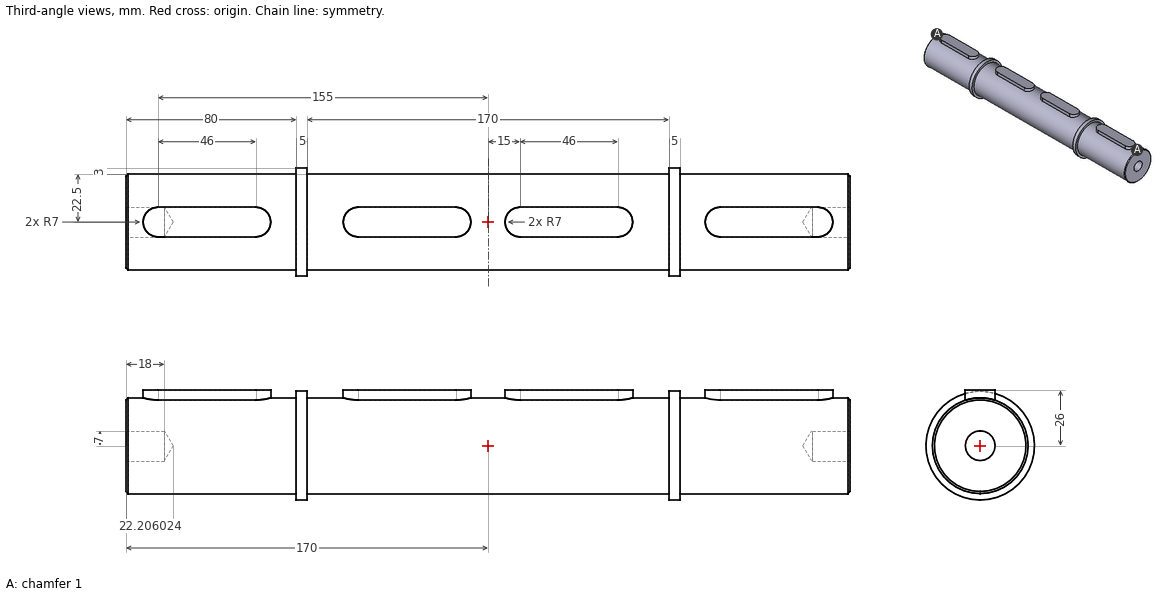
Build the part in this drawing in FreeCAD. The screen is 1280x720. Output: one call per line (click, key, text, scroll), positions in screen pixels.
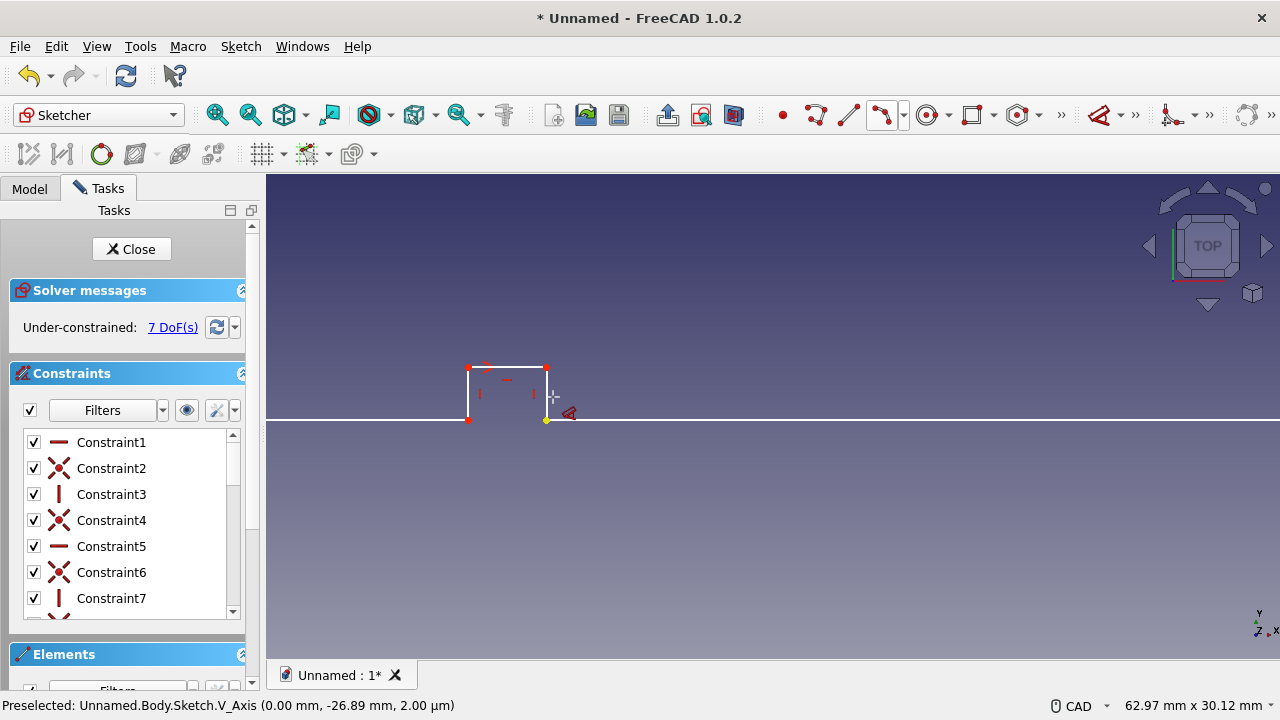
click(547, 394)
click(513, 394)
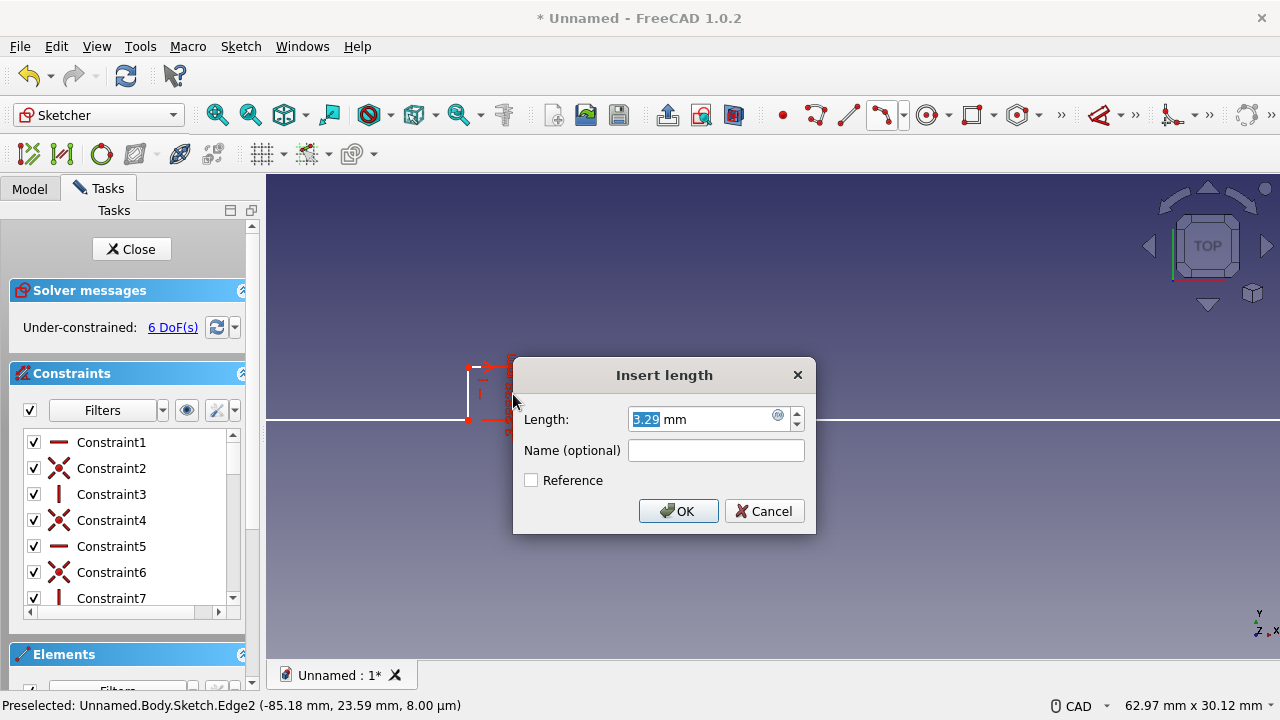
text(3)
key(Return)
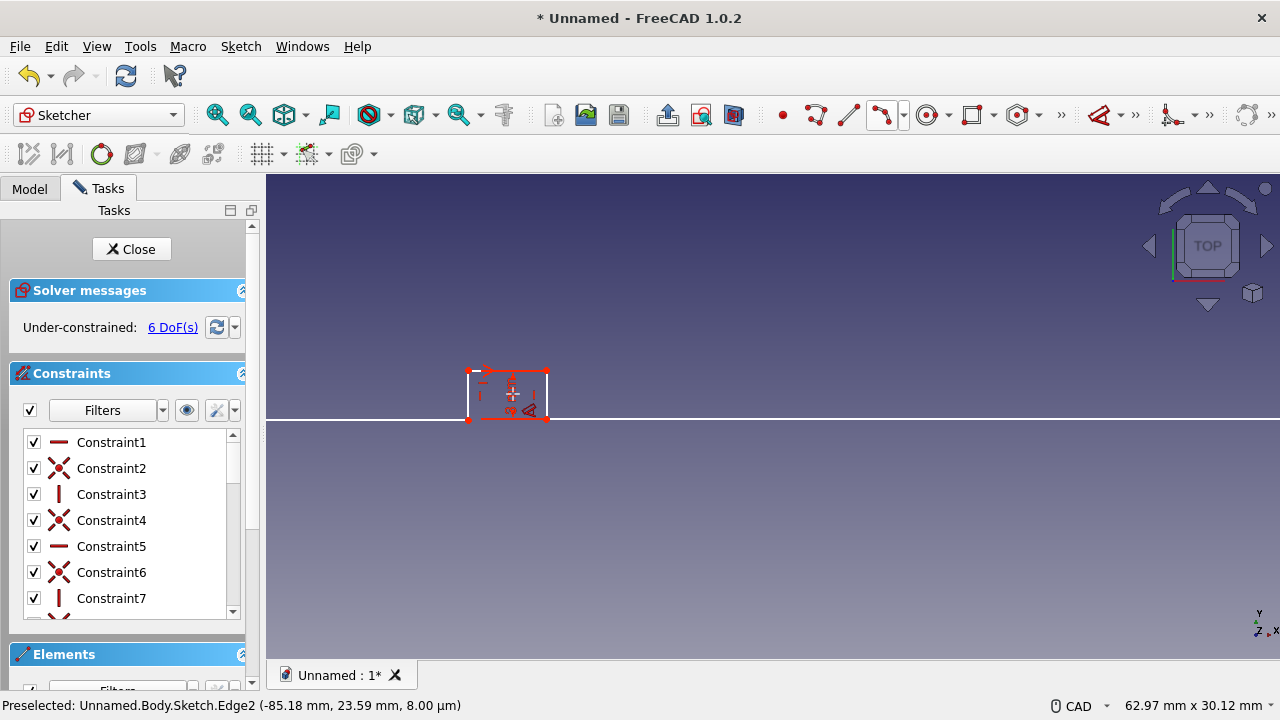
click(523, 371)
click(508, 337)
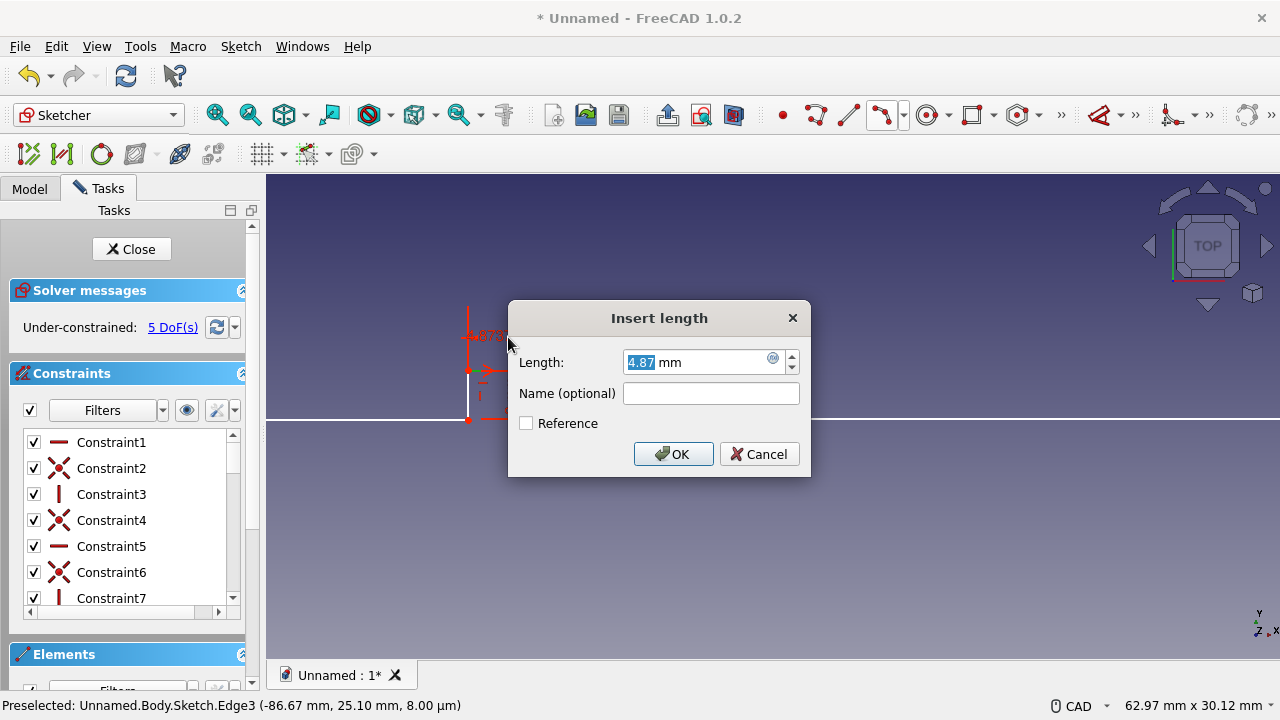
text(5)
key(Return)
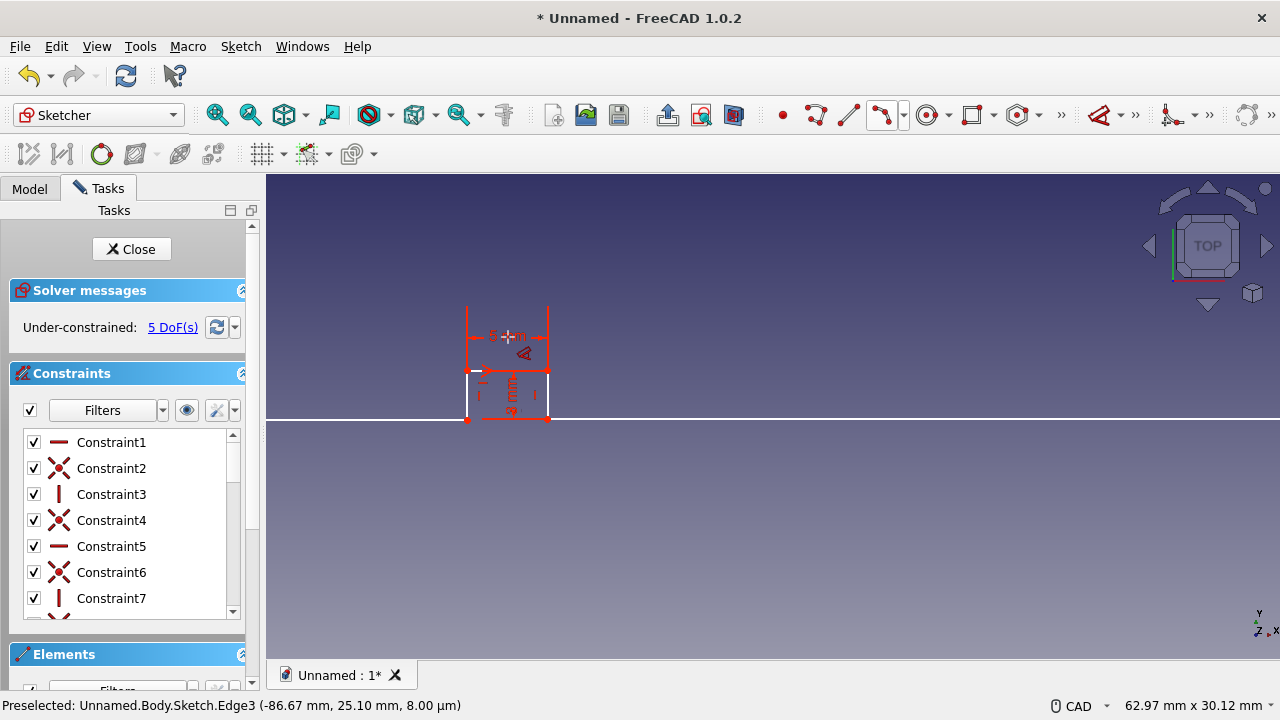
click(467, 386)
click(433, 395)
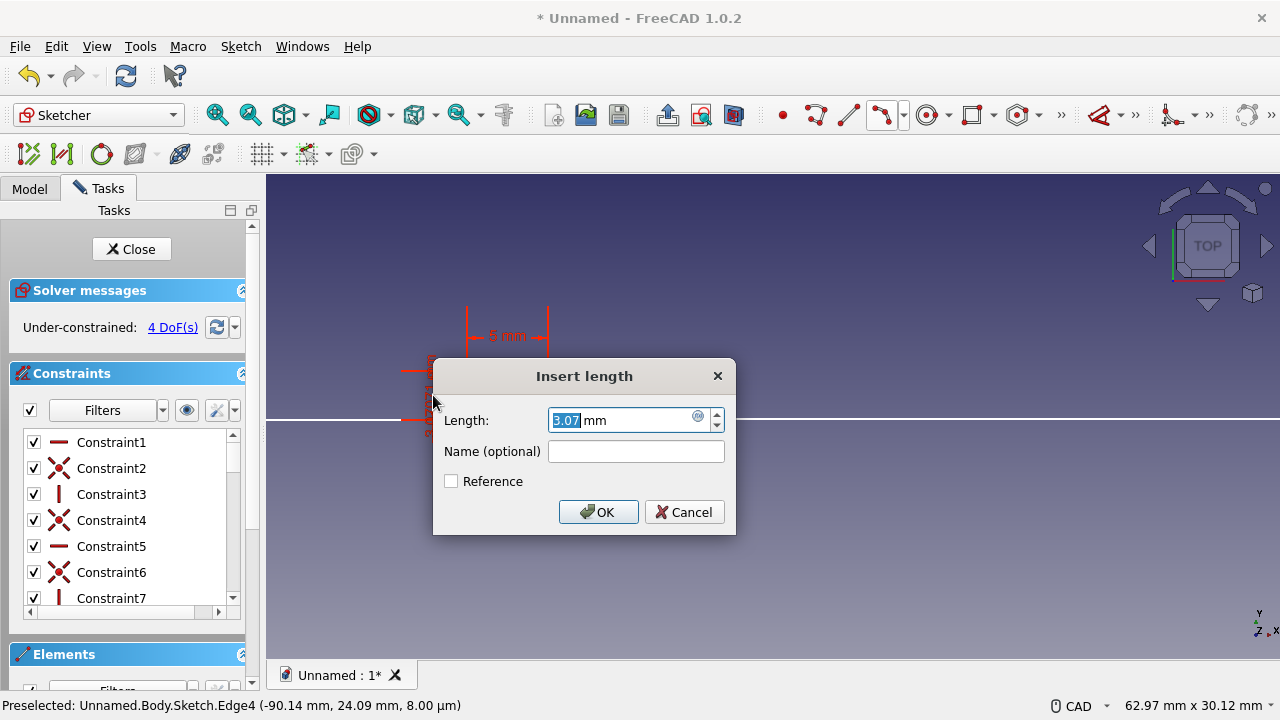
text(3)
key(Return)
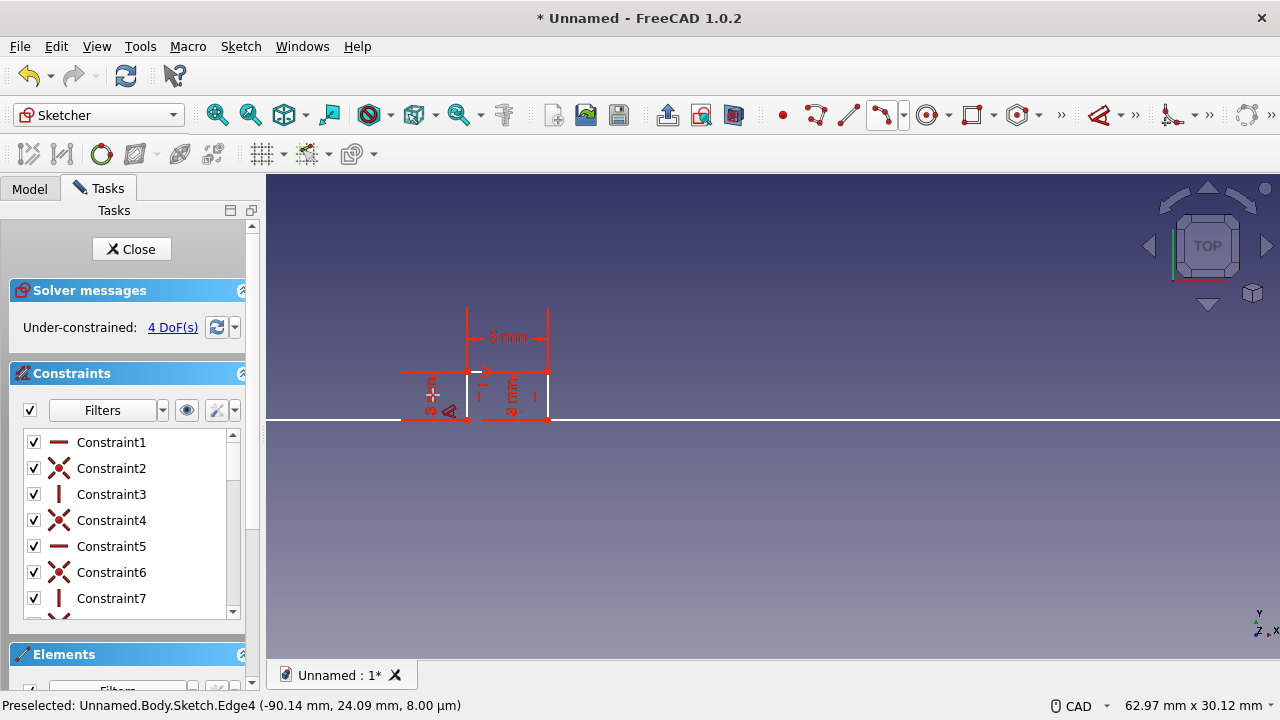
scroll(553, 397, down, 11)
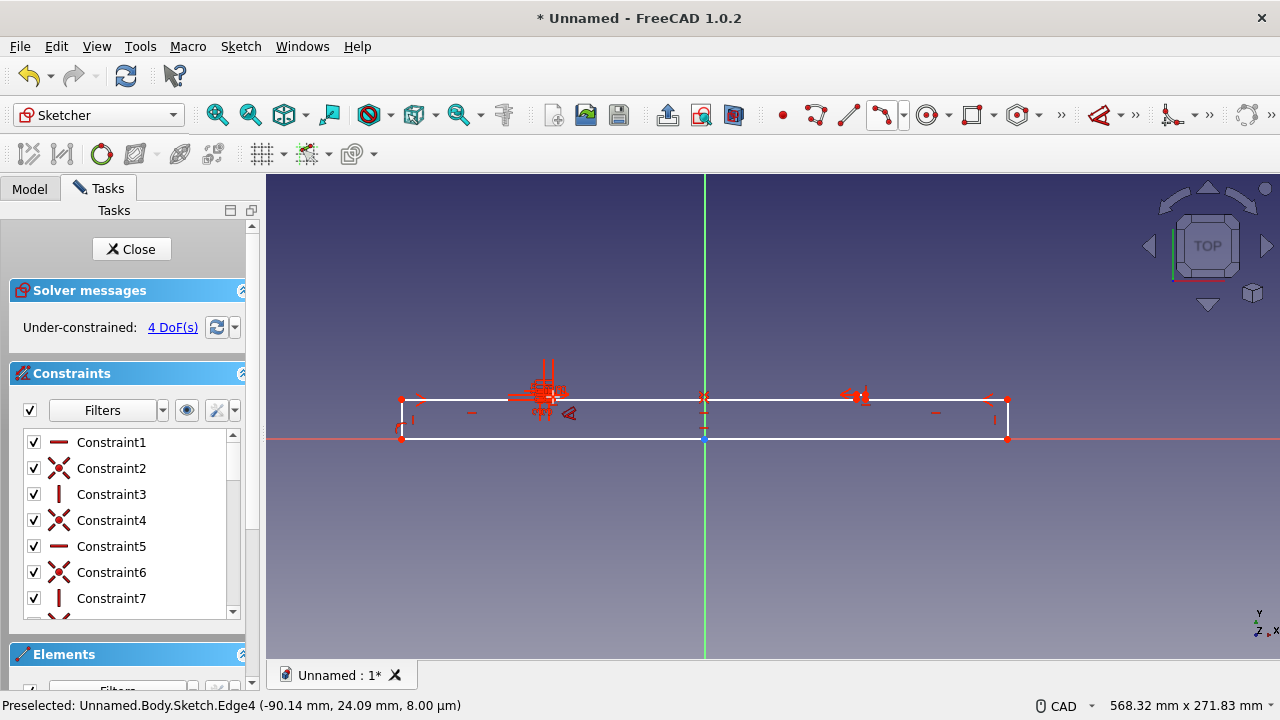
scroll(863, 395, up, 9)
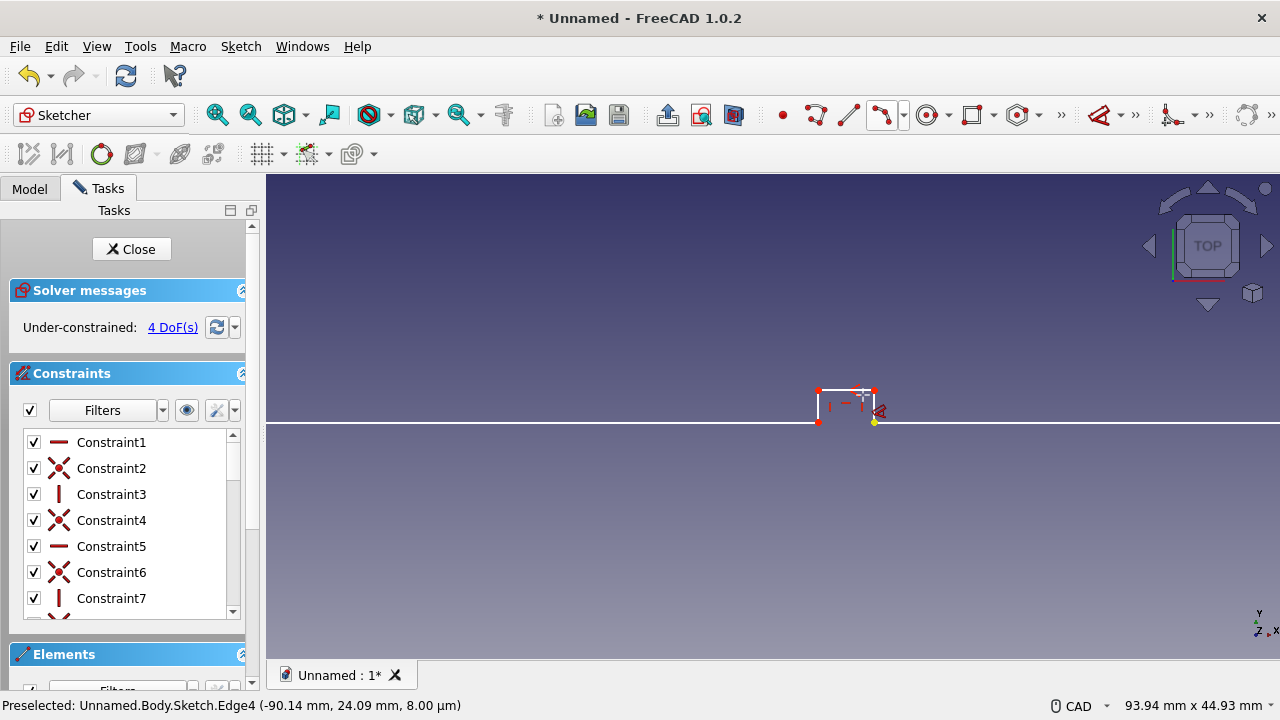
click(858, 390)
click(846, 356)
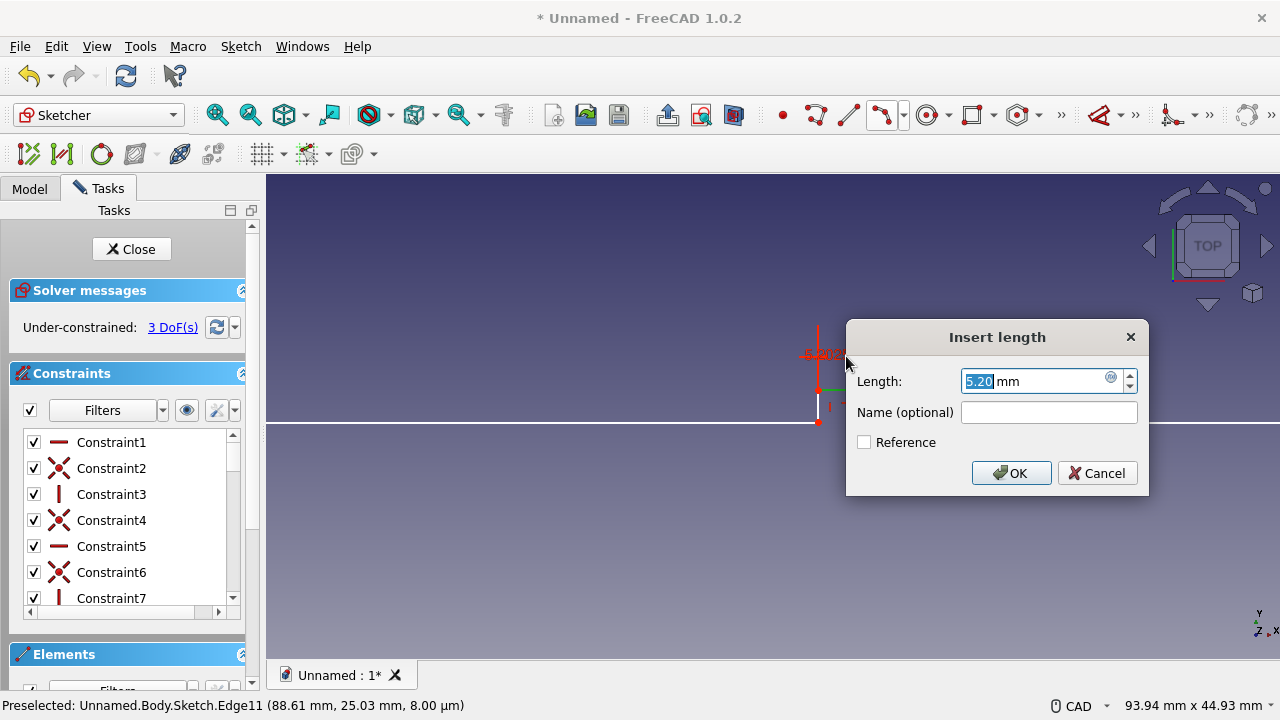
text(5)
key(Return)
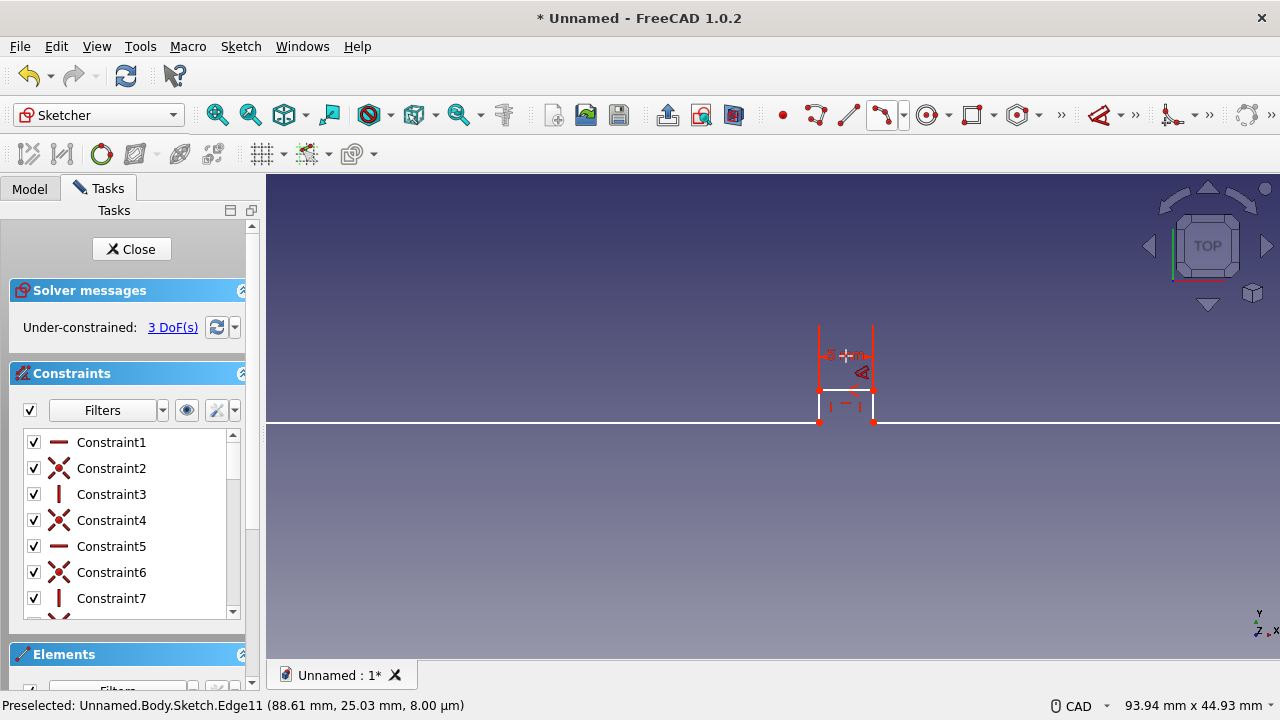
scroll(864, 395, down, 9)